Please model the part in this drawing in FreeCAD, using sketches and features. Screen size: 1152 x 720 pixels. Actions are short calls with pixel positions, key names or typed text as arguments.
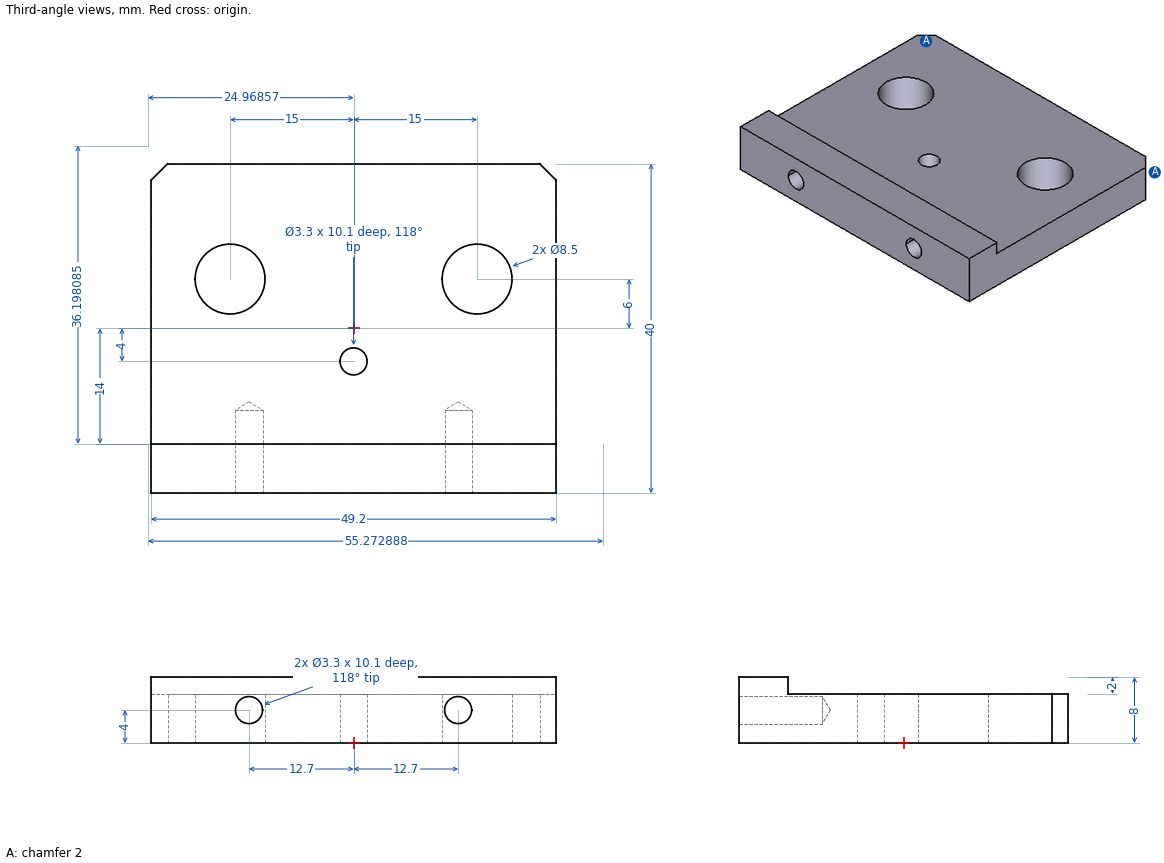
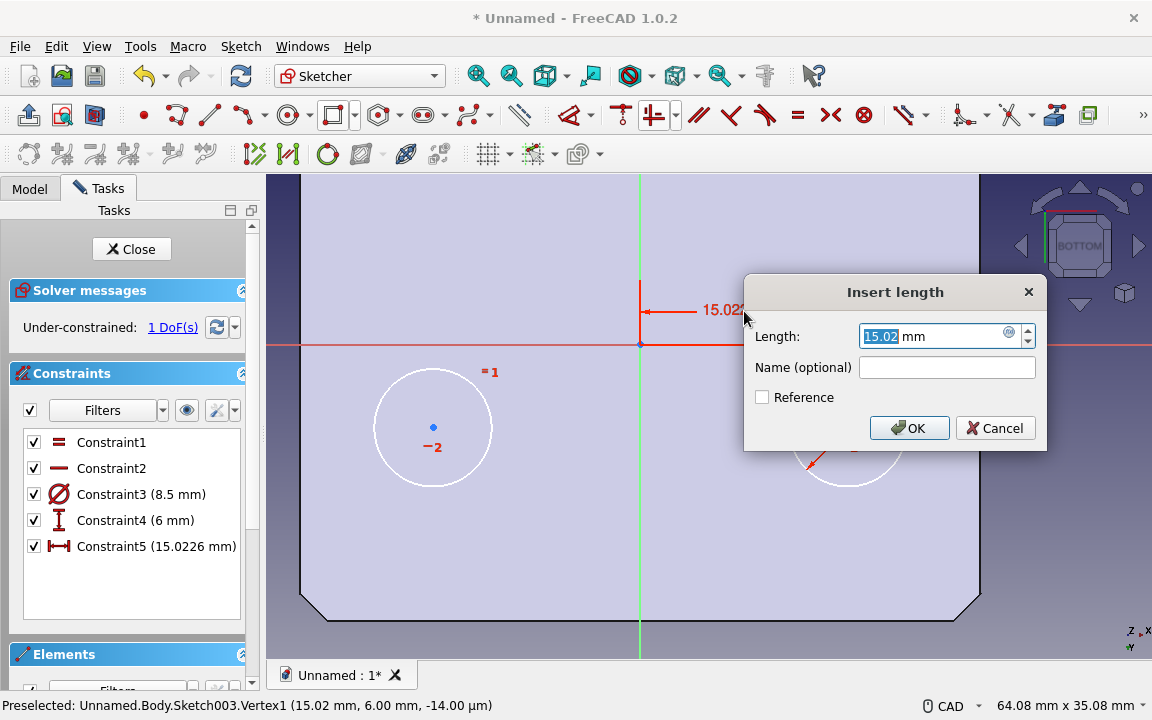
text(15)
key(Return)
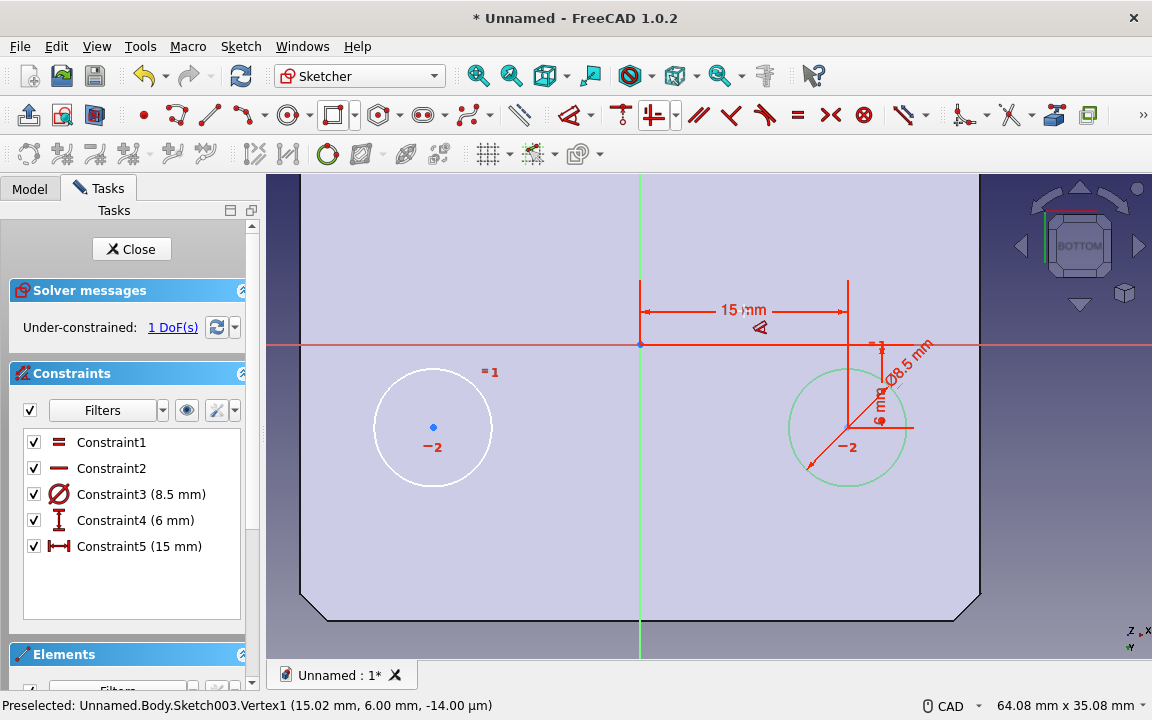
click(433, 428)
click(537, 311)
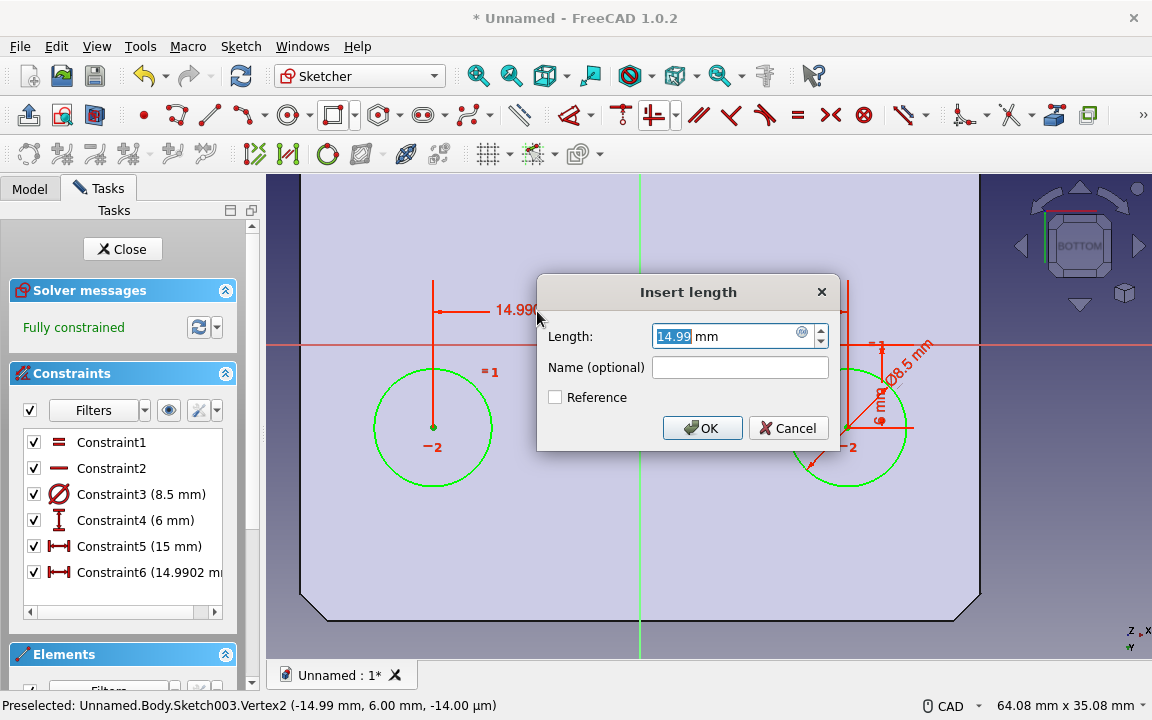
text(15)
key(Return)
key(Escape)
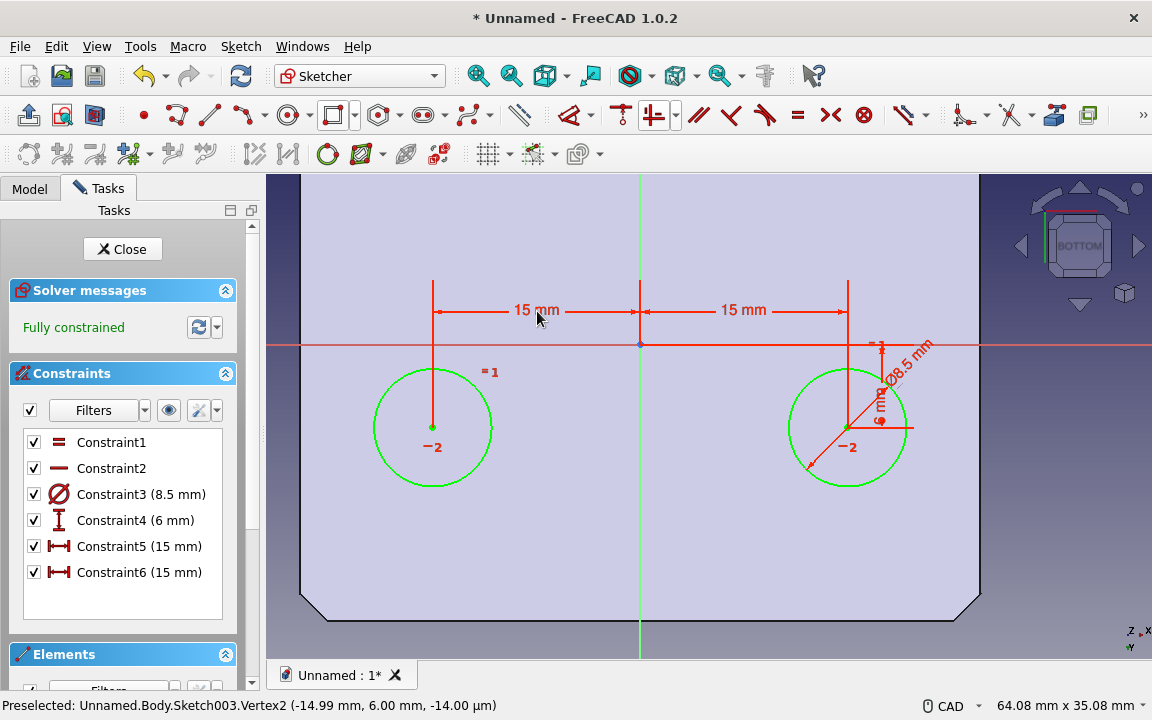
click(123, 249)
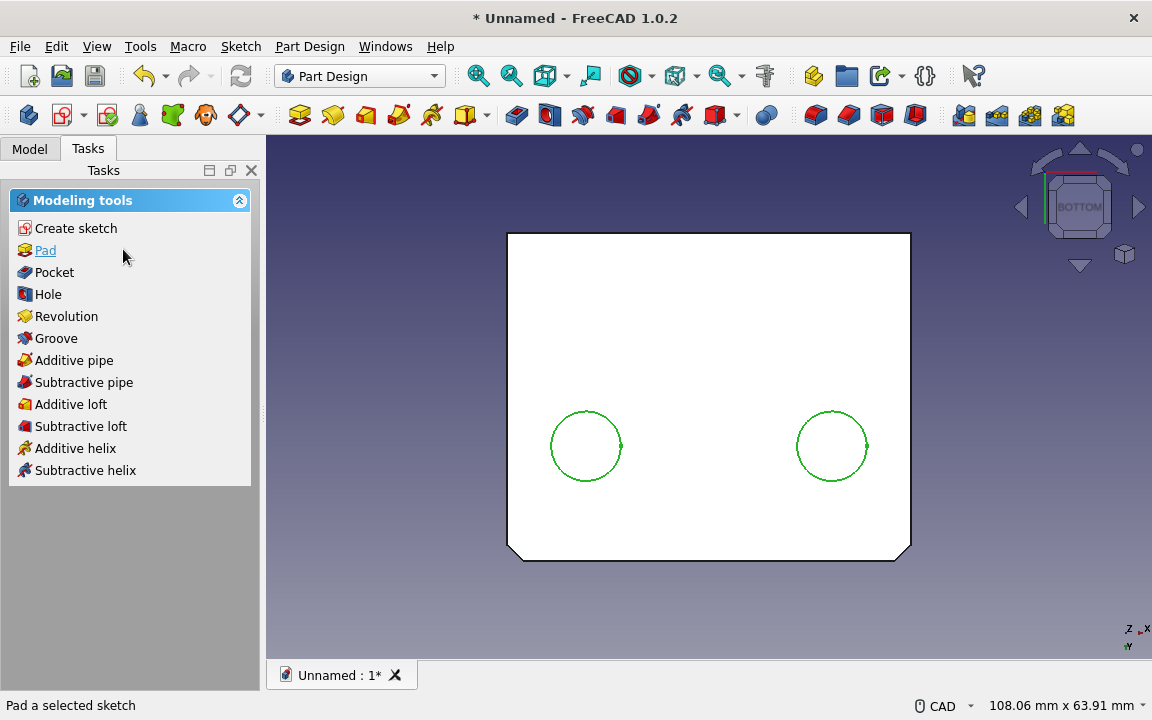
click(517, 116)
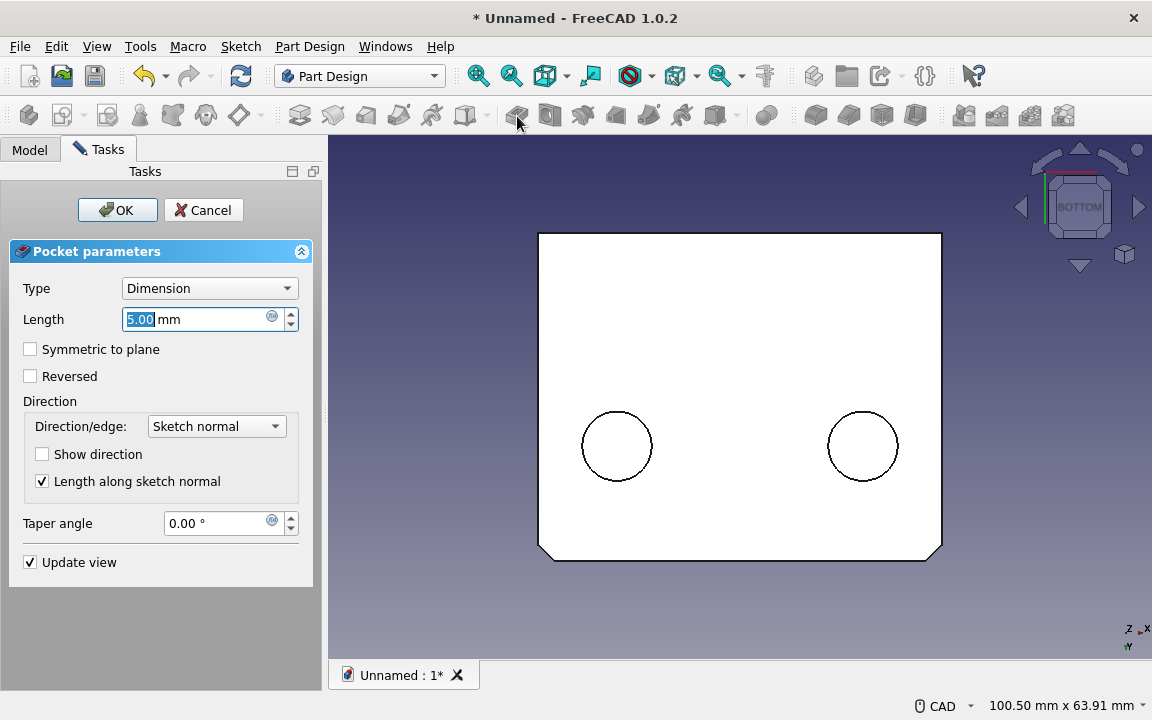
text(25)
key(Tab)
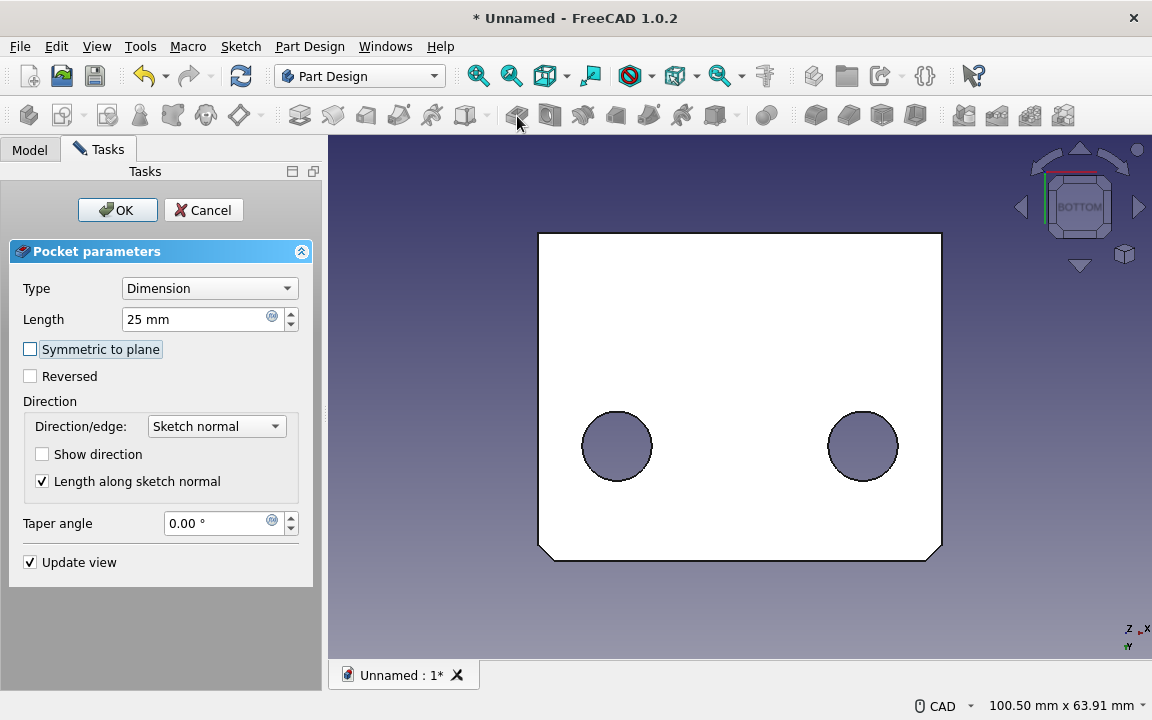
click(118, 210)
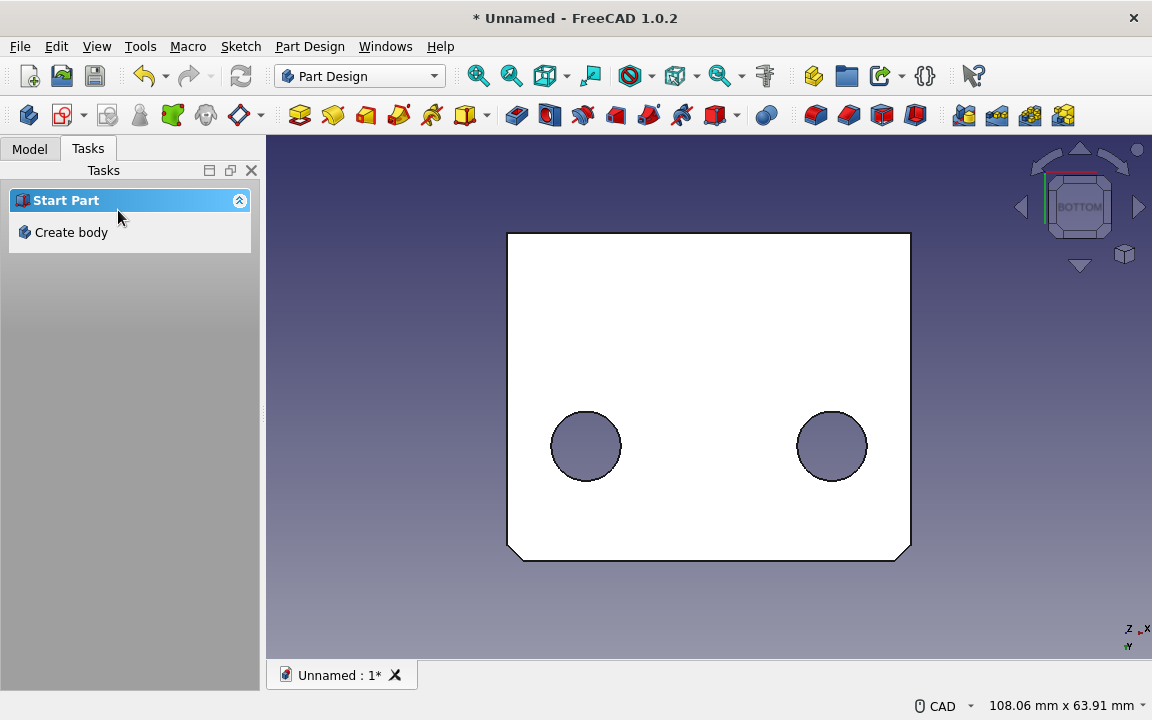
key(0)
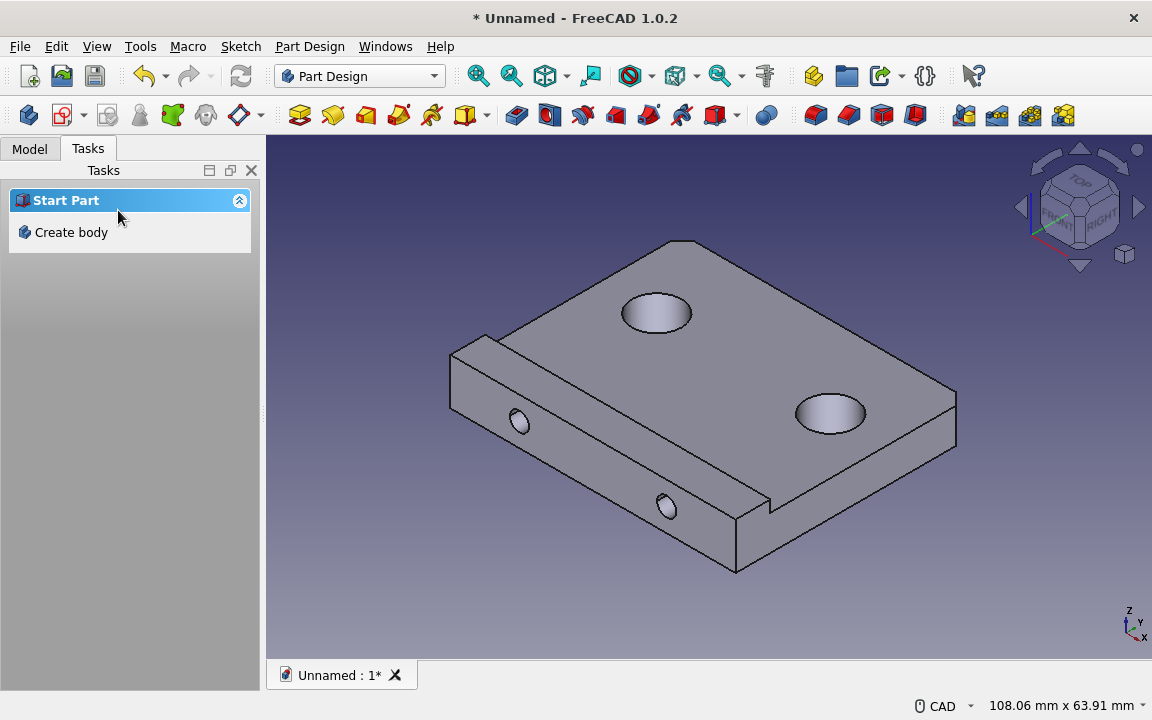
click(698, 389)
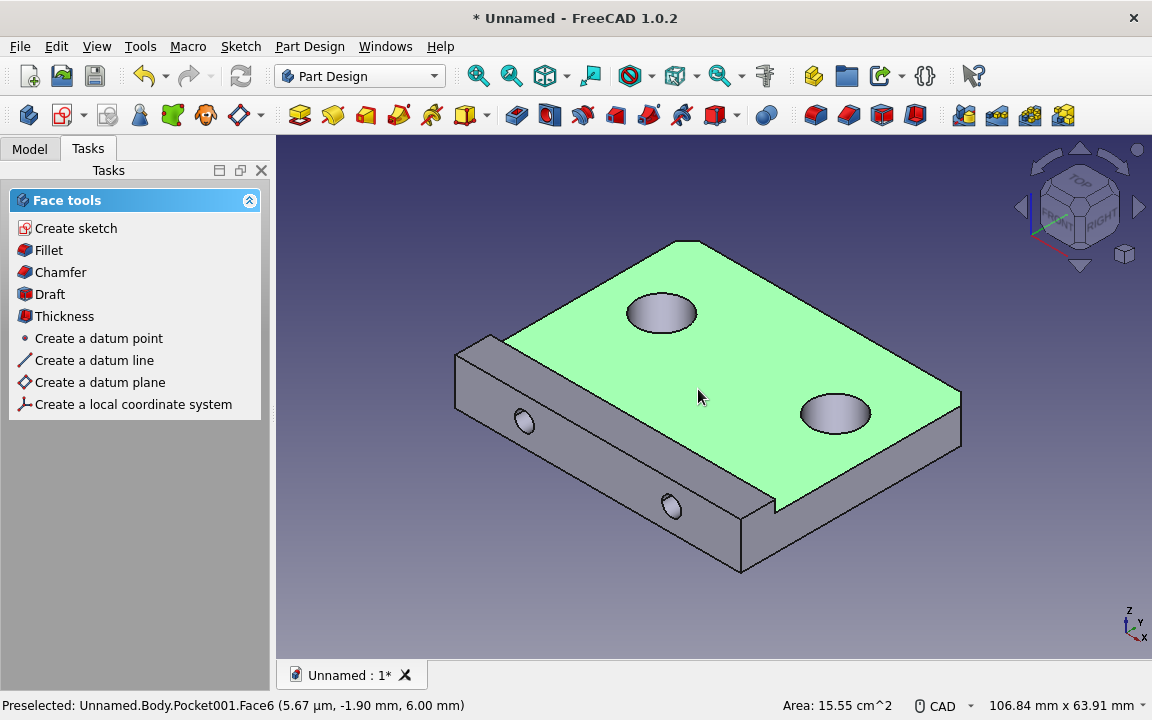
click(62, 116)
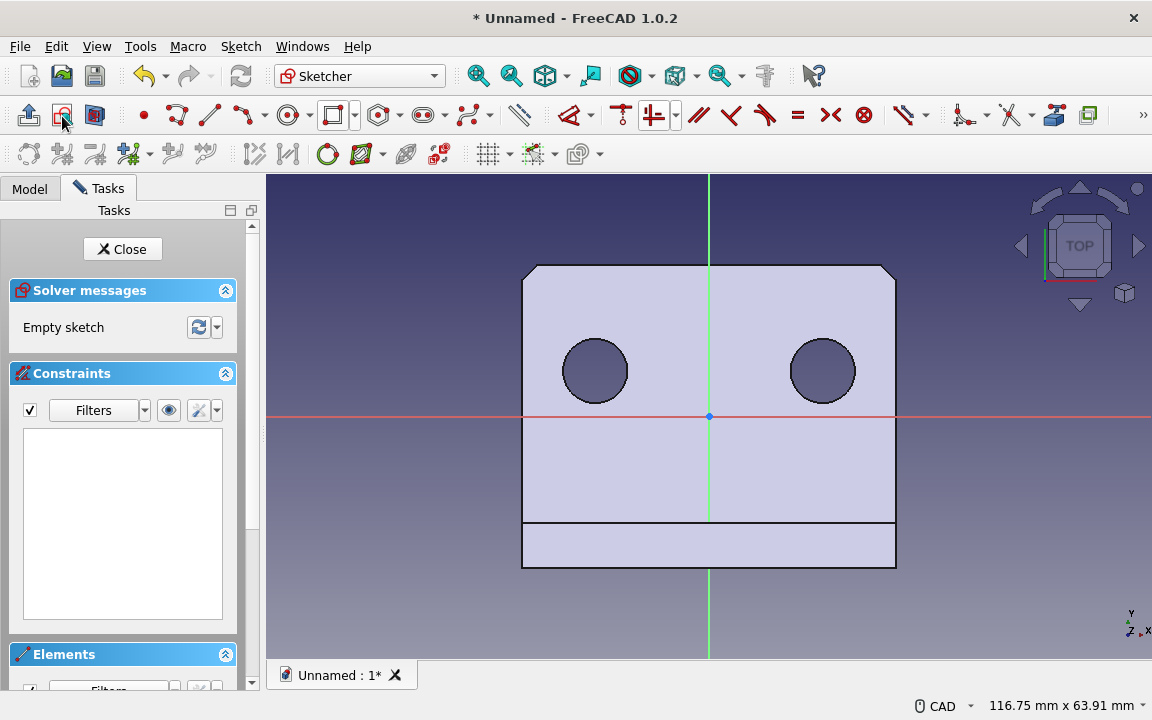
click(95, 116)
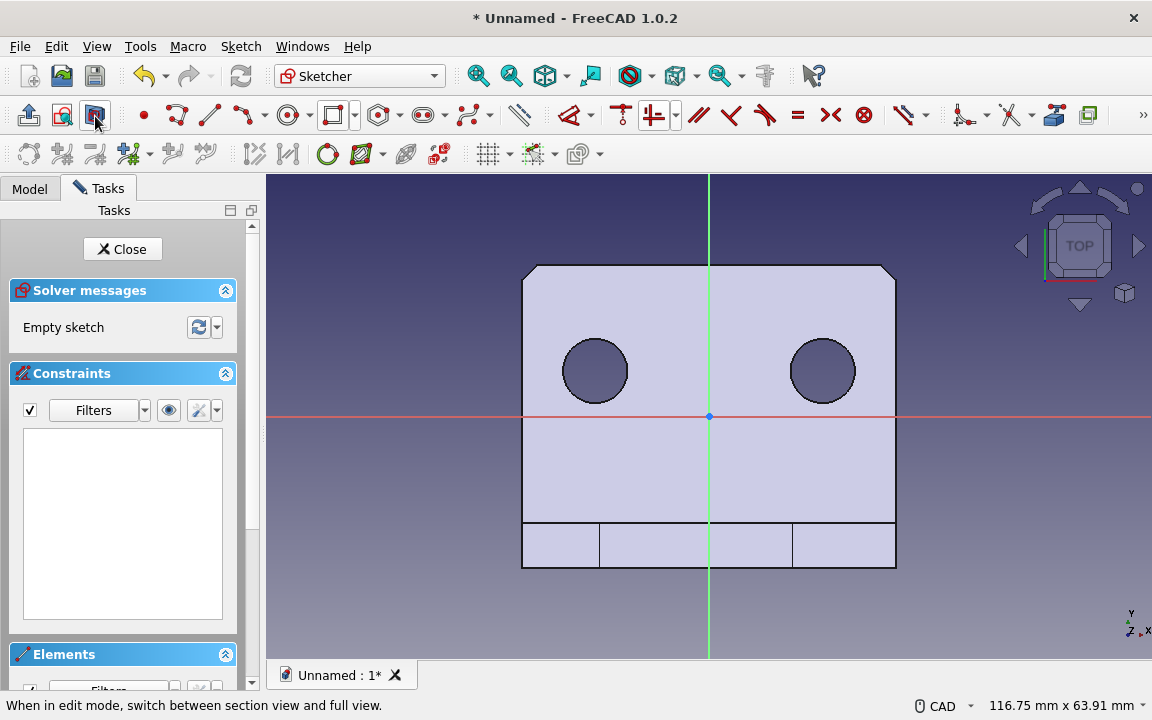
scroll(720, 441, up, 10)